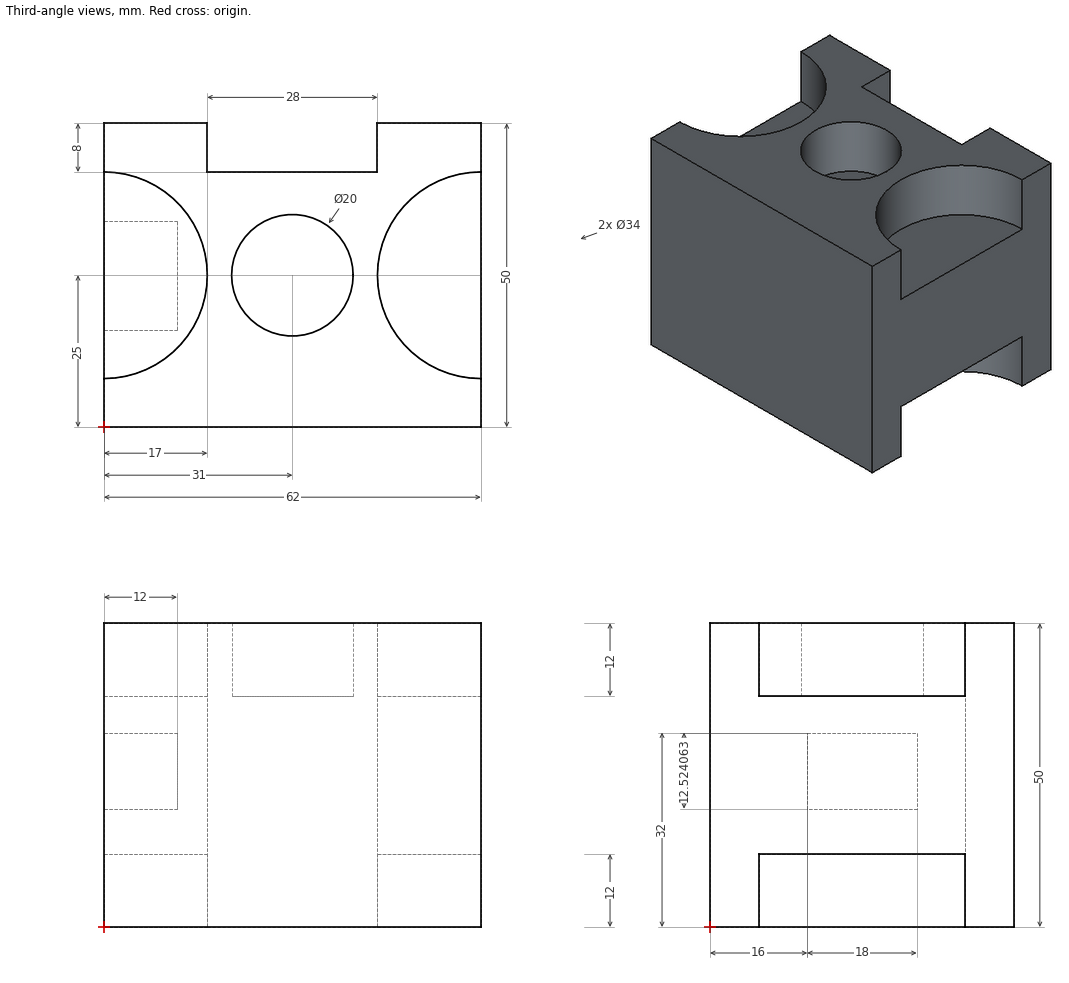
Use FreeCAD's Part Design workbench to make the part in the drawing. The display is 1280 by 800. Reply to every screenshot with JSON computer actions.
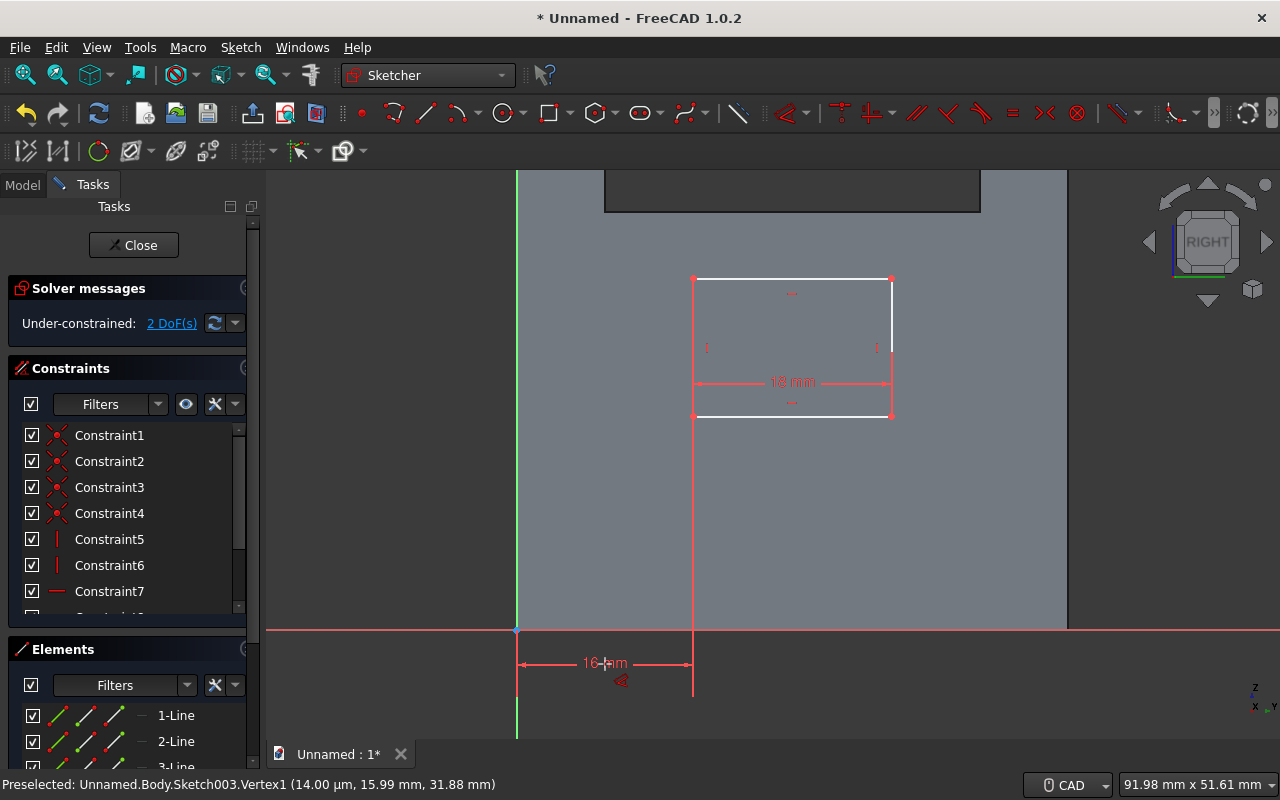
{"action": "left_click", "coordinate": [693, 279]}
{"action": "left_click", "coordinate": [483, 455]}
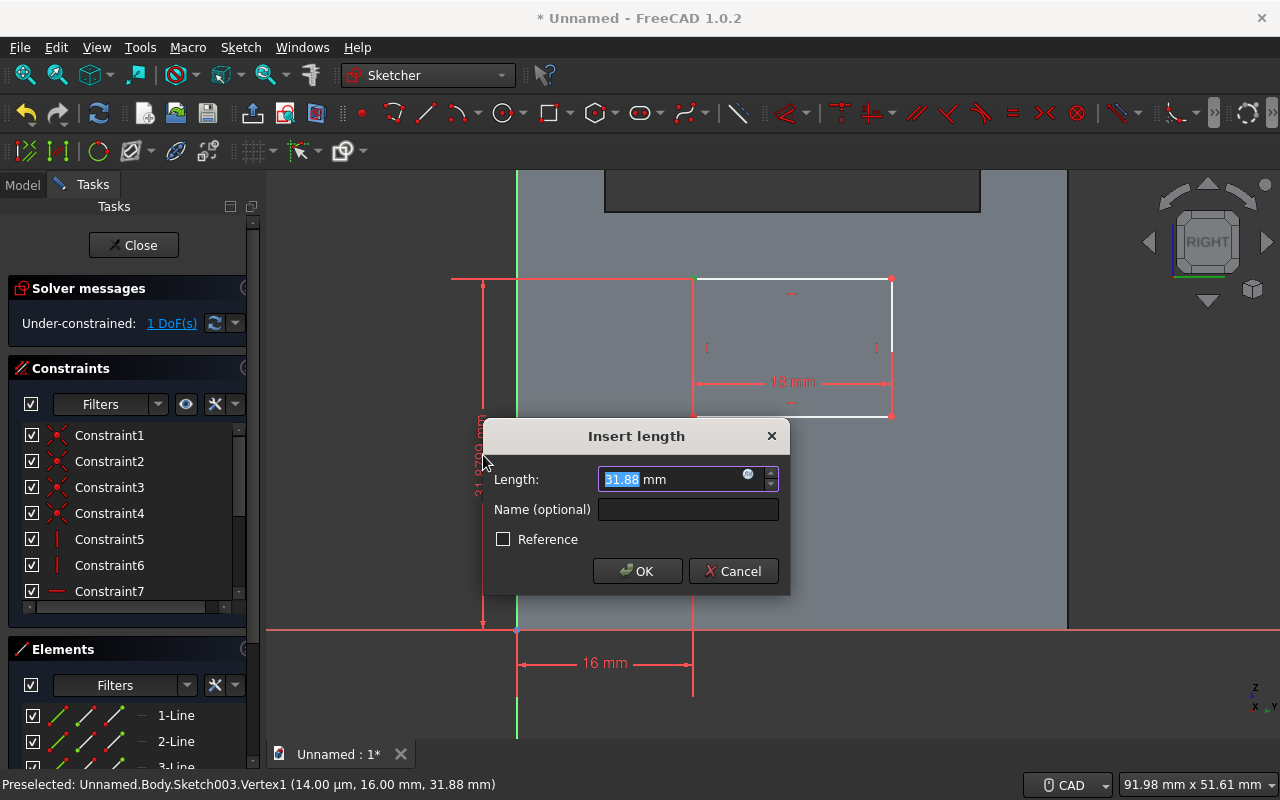
{"action": "type", "text": "32"}
{"action": "key", "text": "Return"}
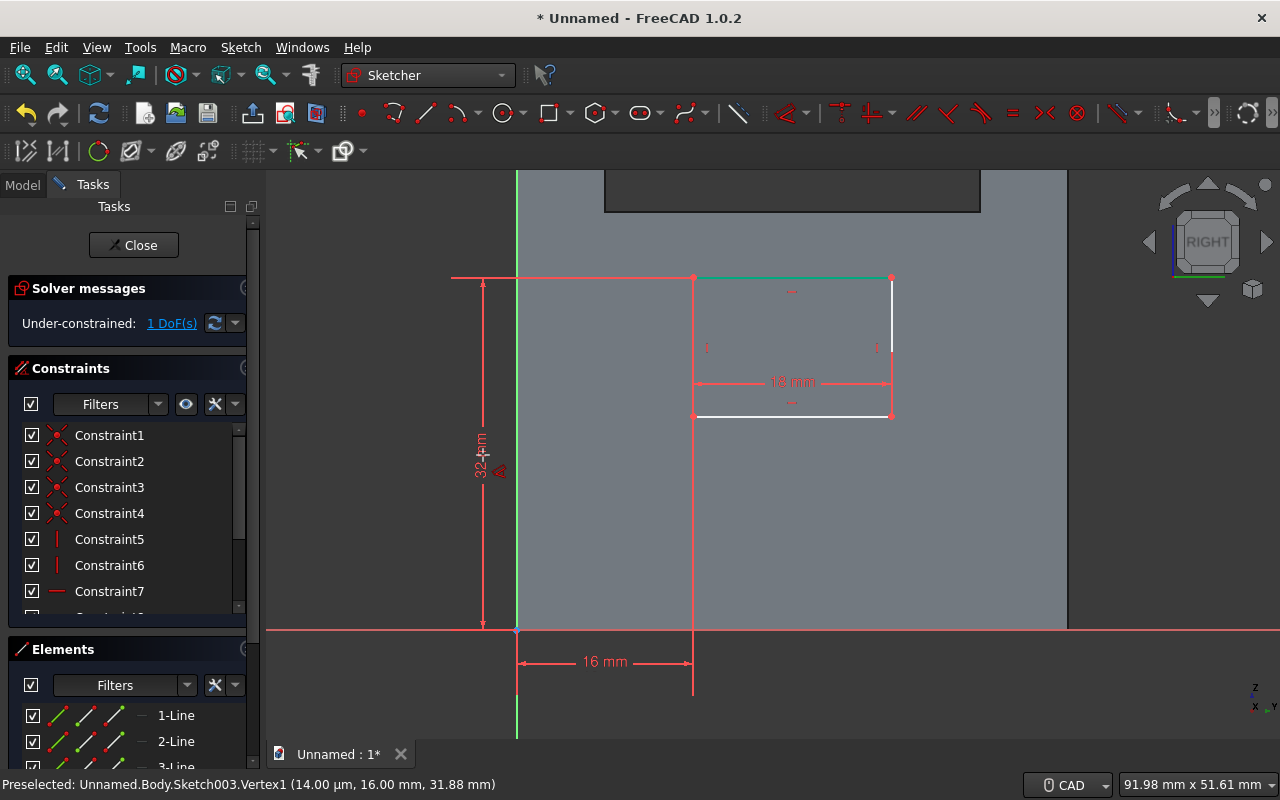
{"action": "left_click", "coordinate": [693, 319]}
{"action": "left_click", "coordinate": [659, 347]}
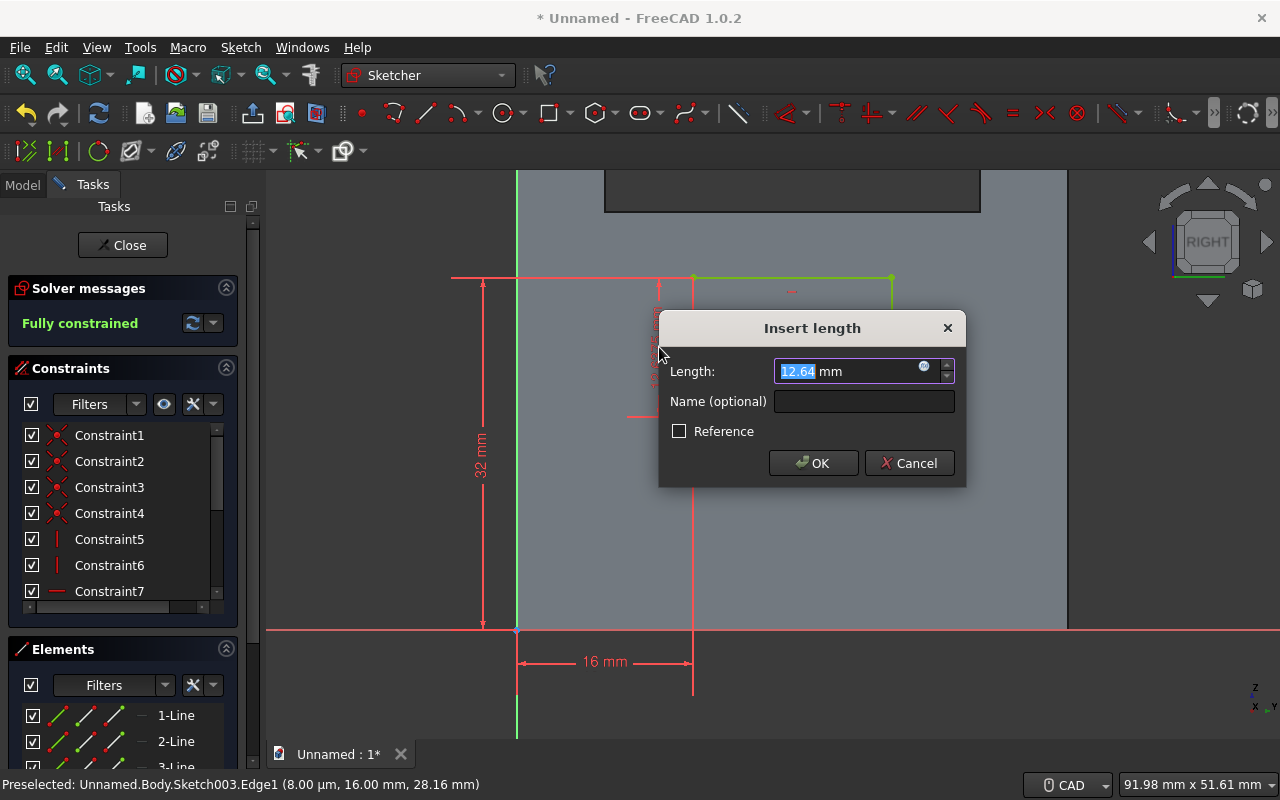
{"action": "type", "text": "12.524063"}
{"action": "key", "text": "Return"}
{"action": "key", "text": "Escape"}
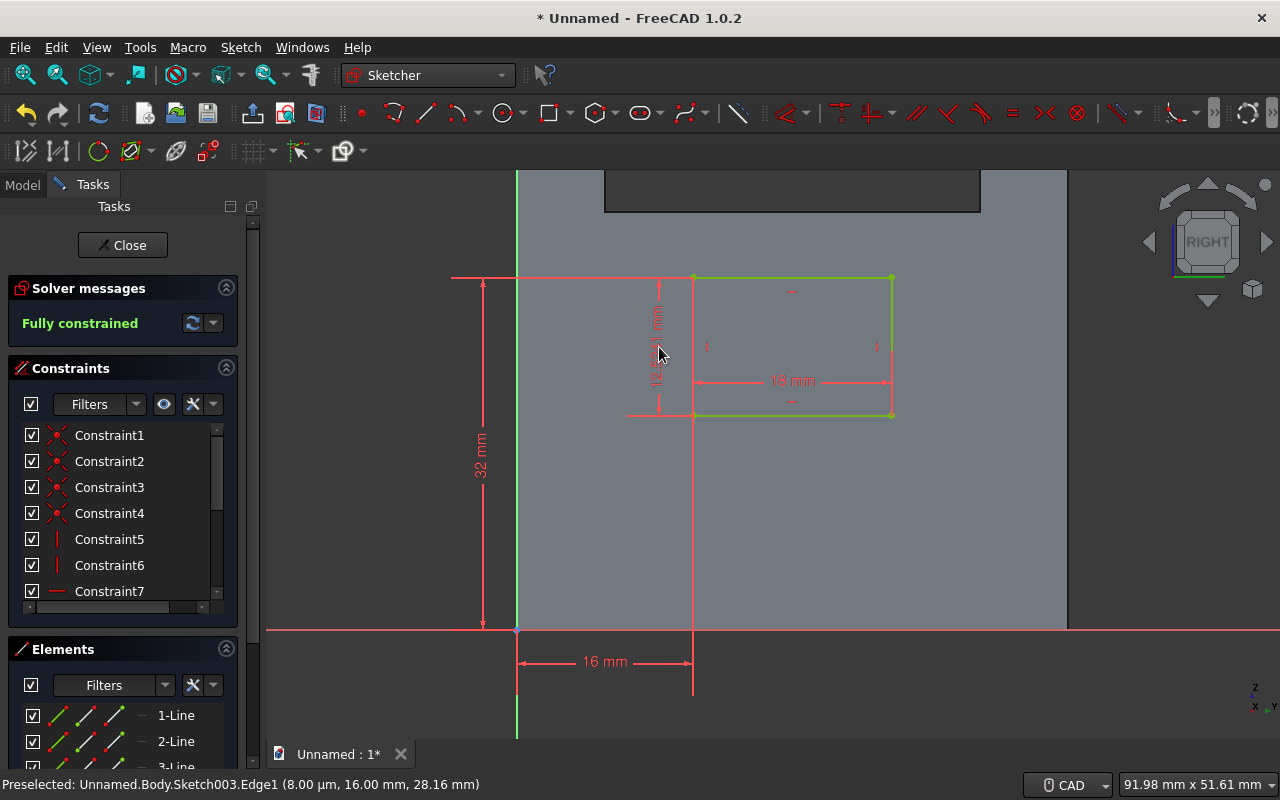
{"action": "left_click", "coordinate": [123, 245]}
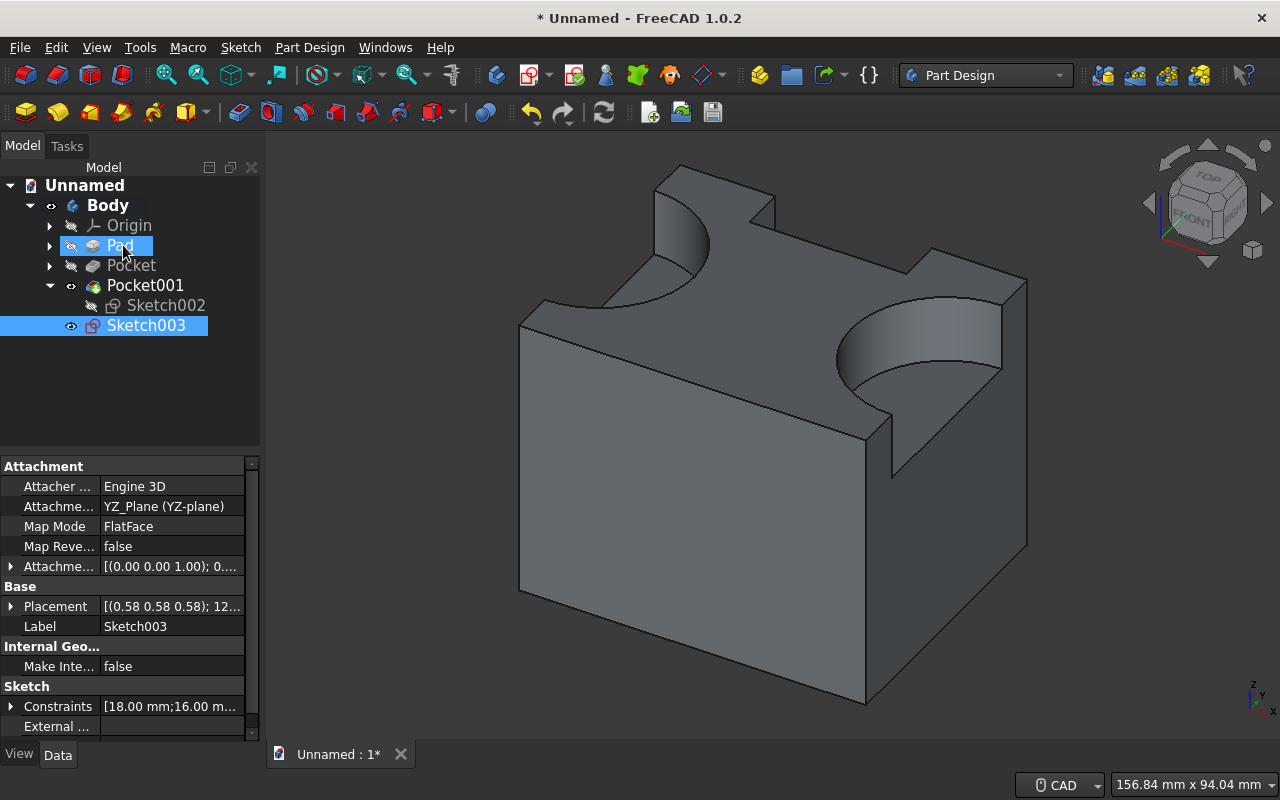
{"action": "left_click", "coordinate": [240, 112]}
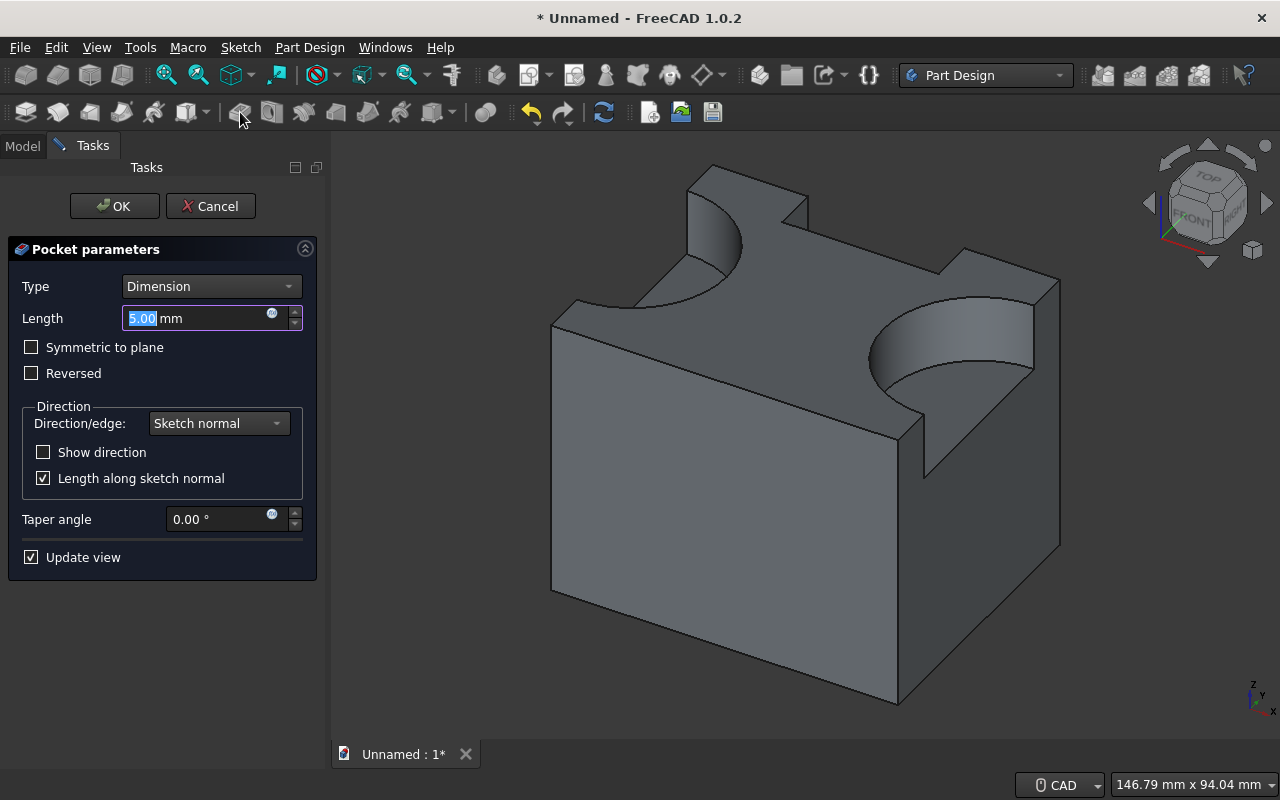
{"action": "type", "text": "12"}
{"action": "key", "text": "Tab"}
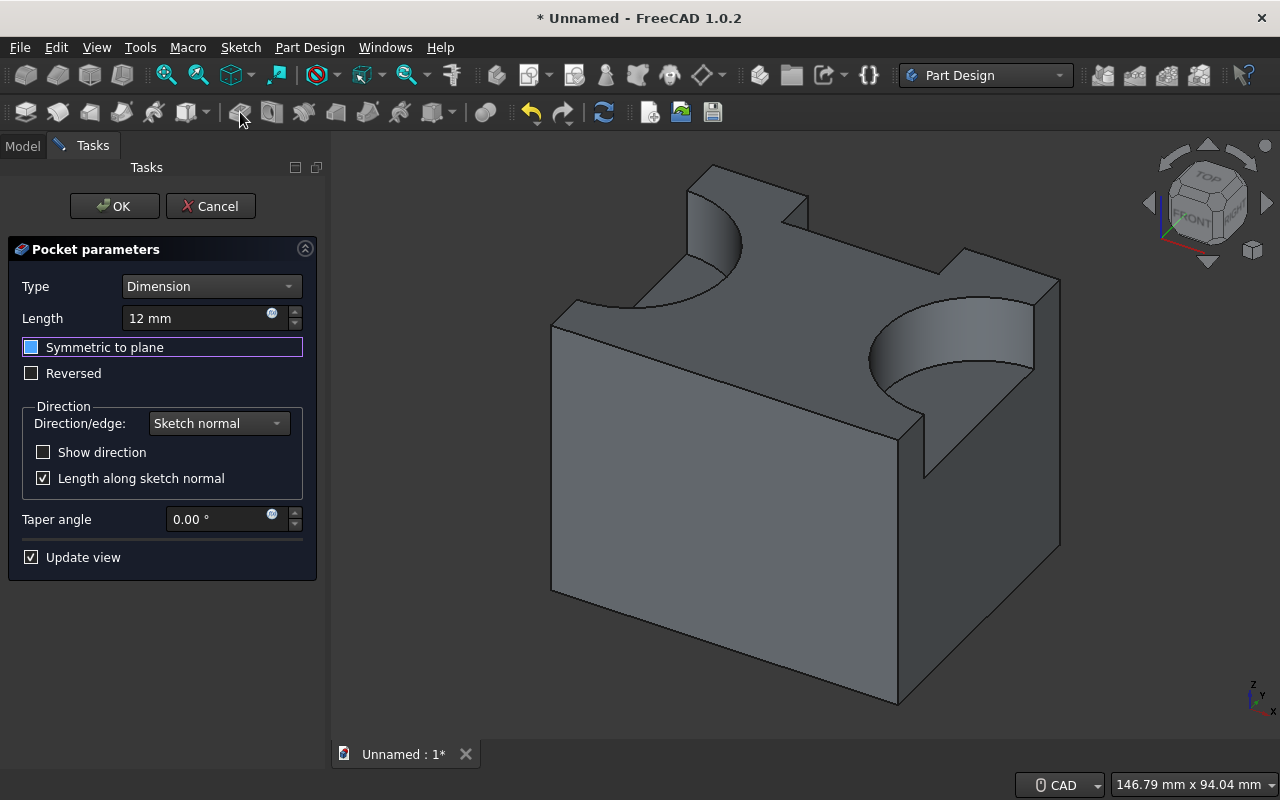
{"action": "left_click", "coordinate": [30, 373]}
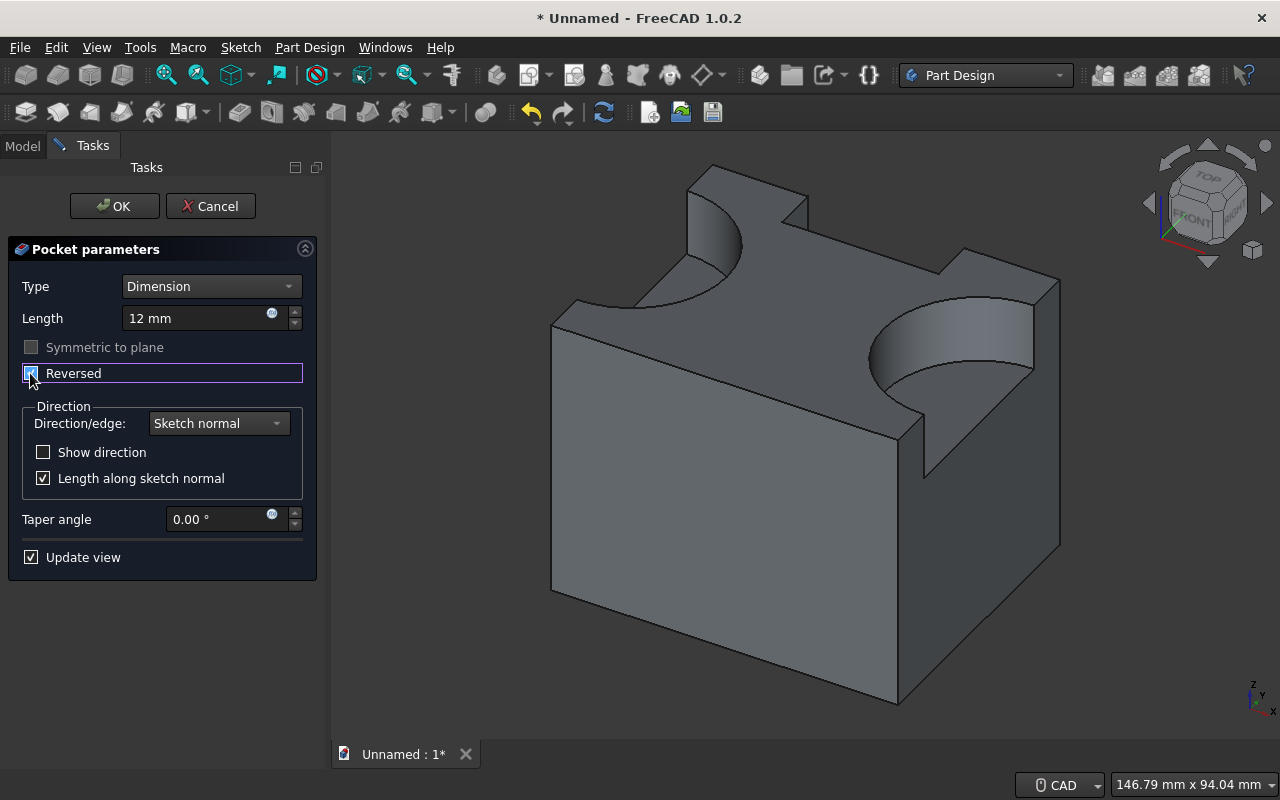
{"action": "left_click", "coordinate": [115, 206]}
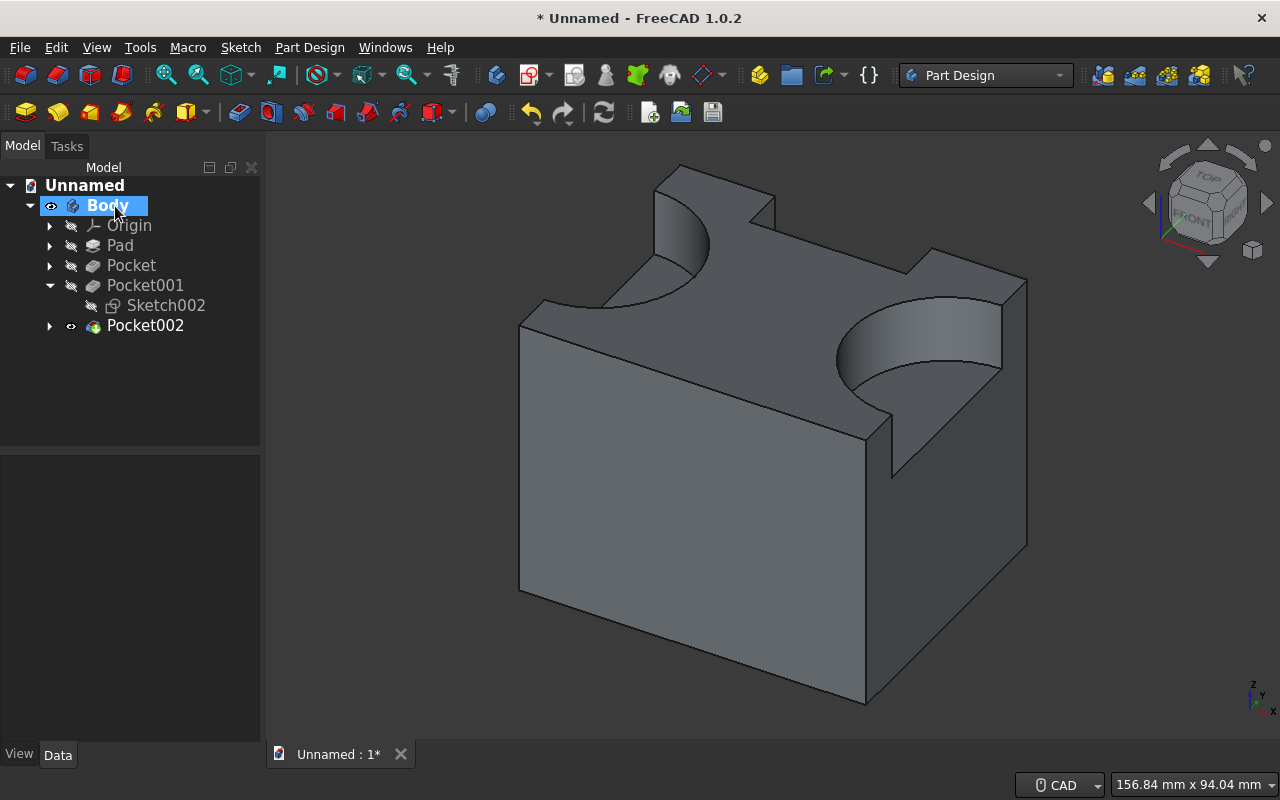
{"action": "left_click", "coordinate": [50, 226]}